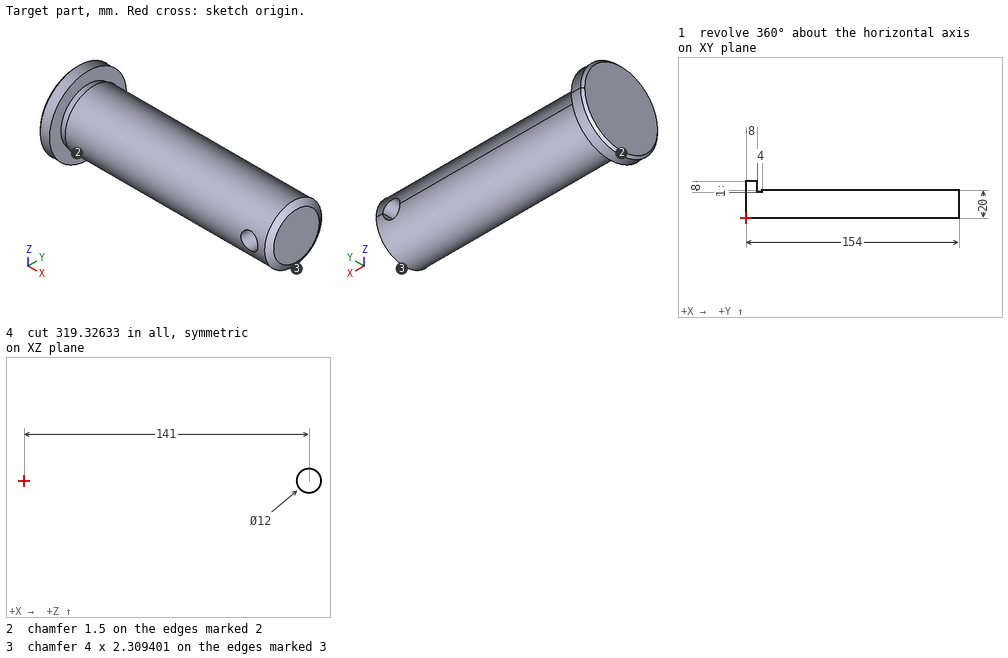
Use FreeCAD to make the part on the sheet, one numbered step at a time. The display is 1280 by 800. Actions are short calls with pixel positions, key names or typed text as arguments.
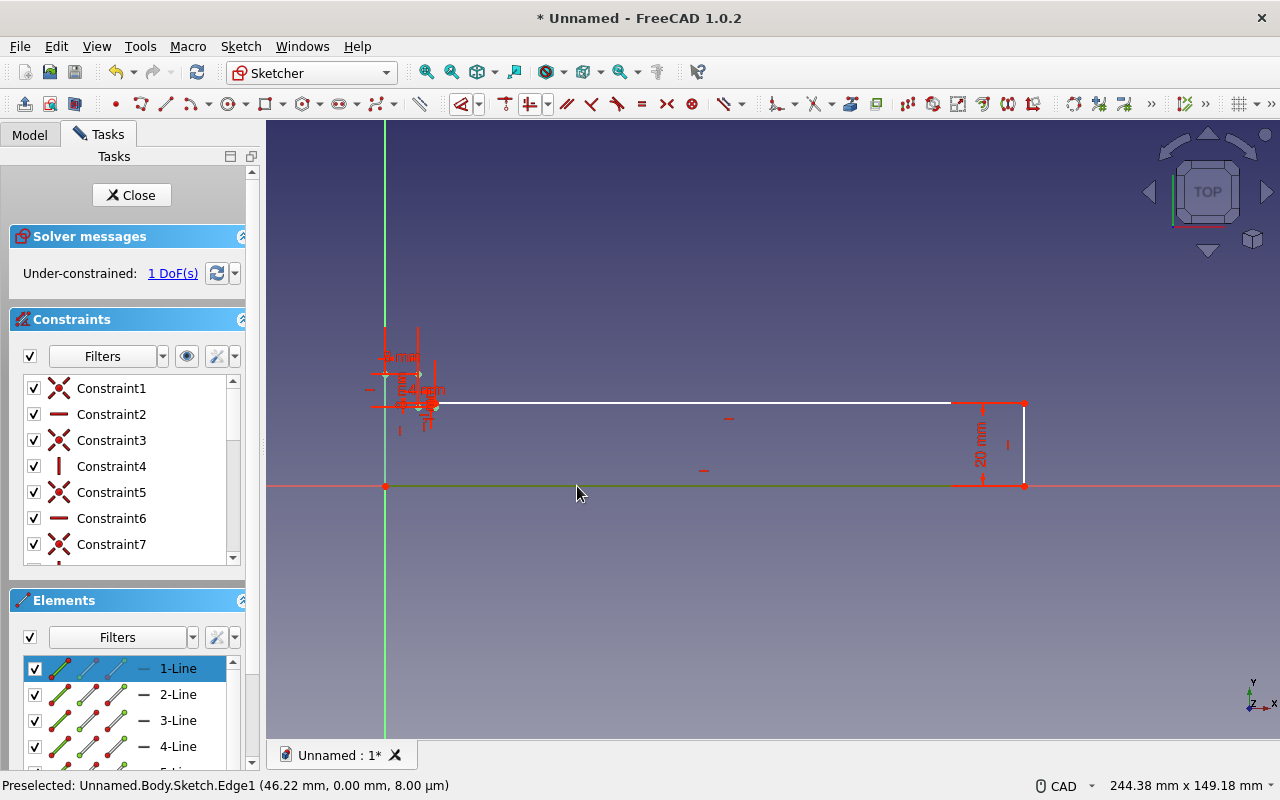
click(478, 104)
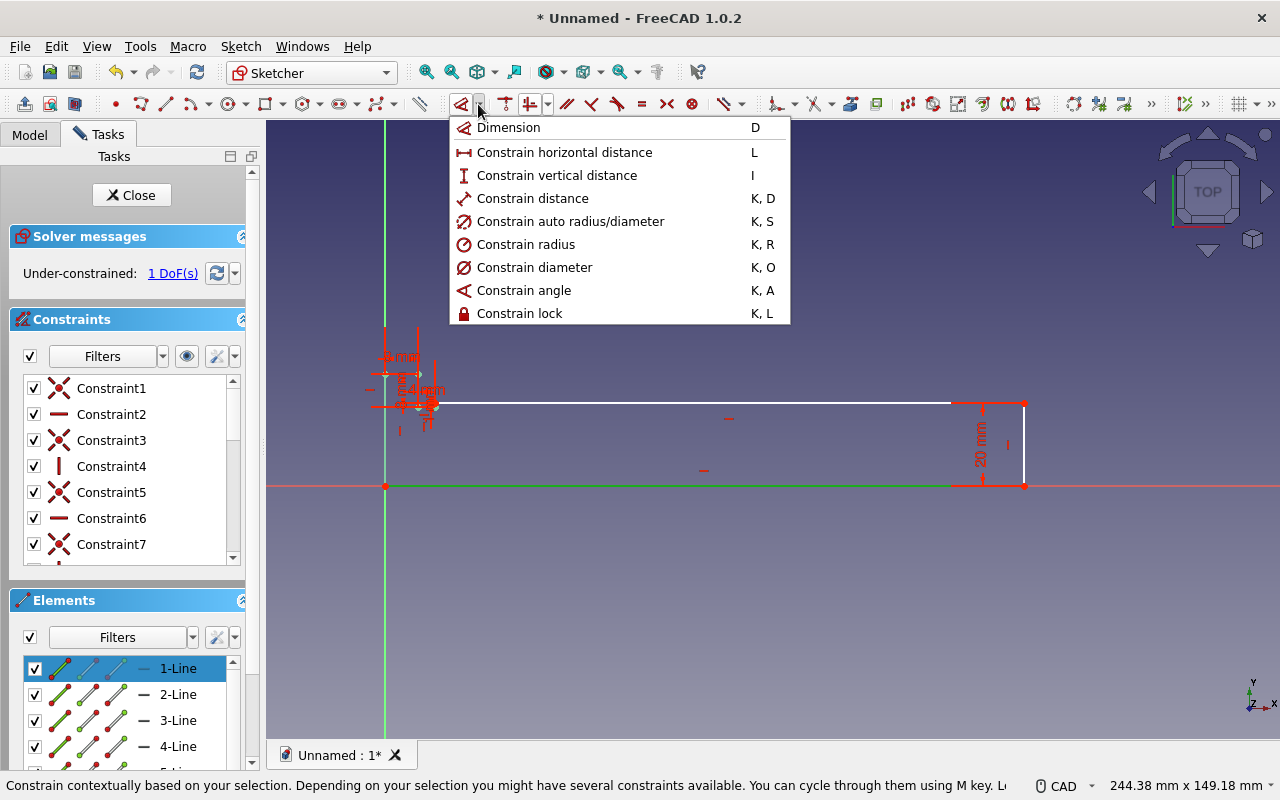
click(620, 152)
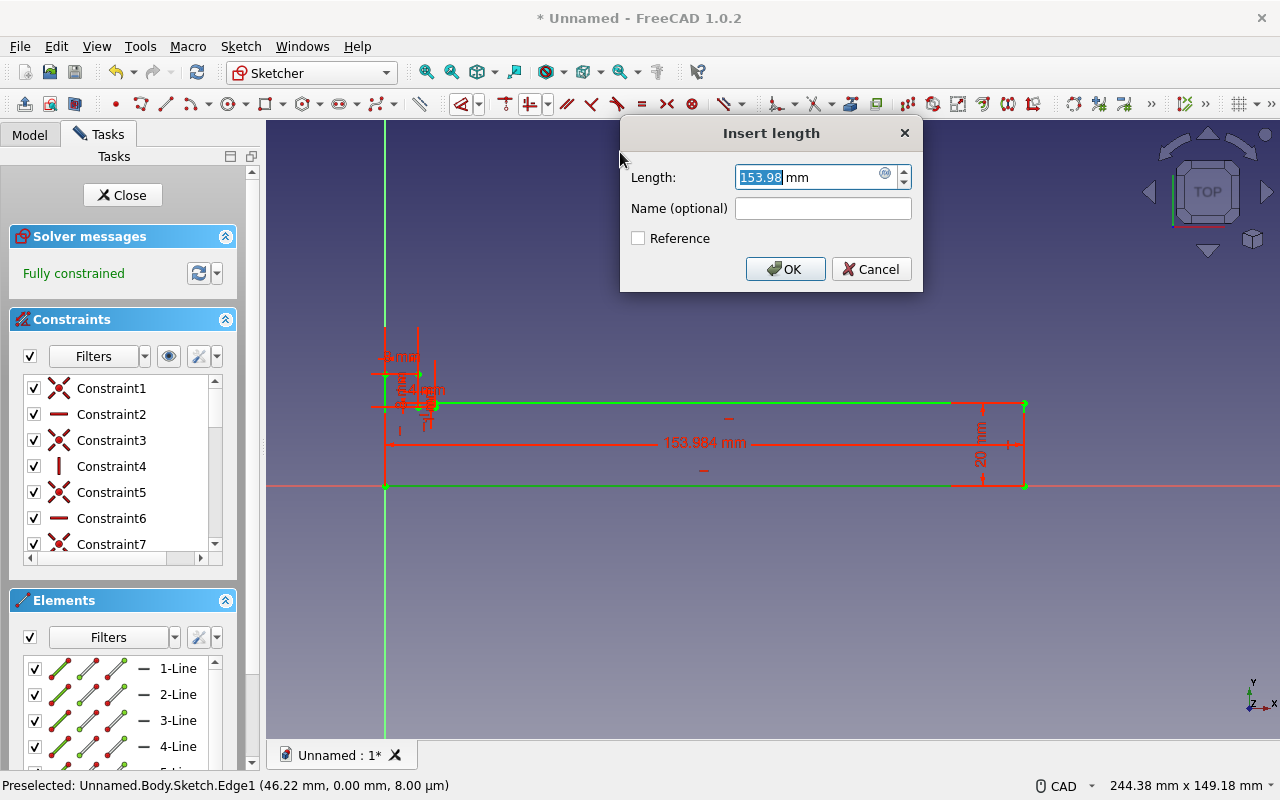
text(154)
key(Return)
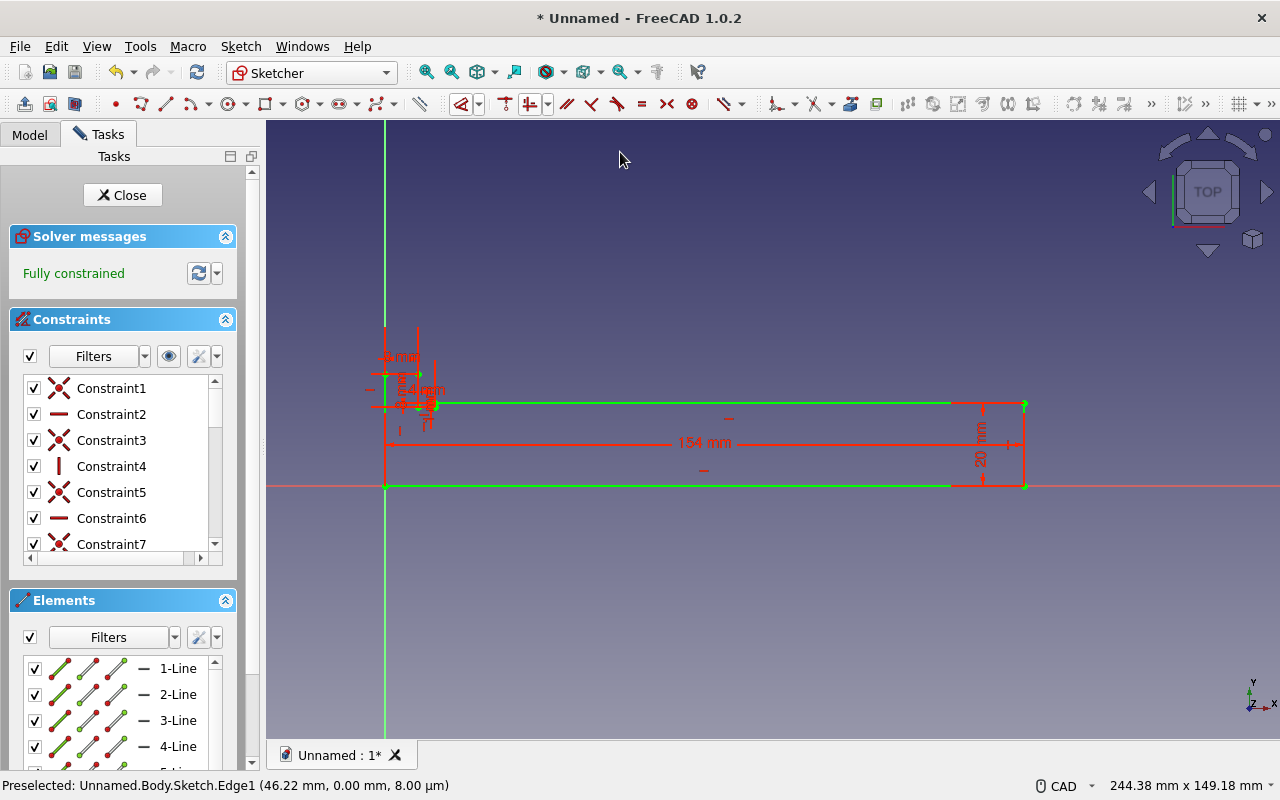
click(123, 195)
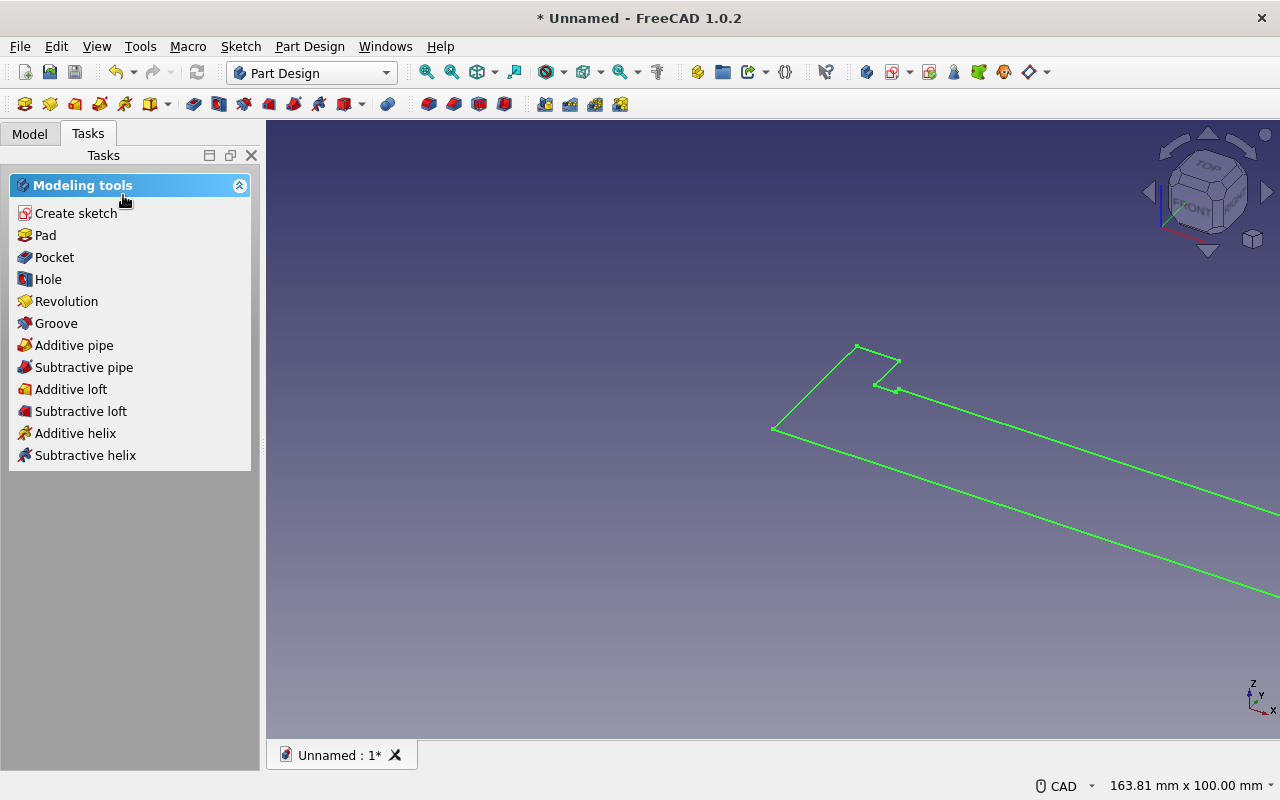
click(50, 104)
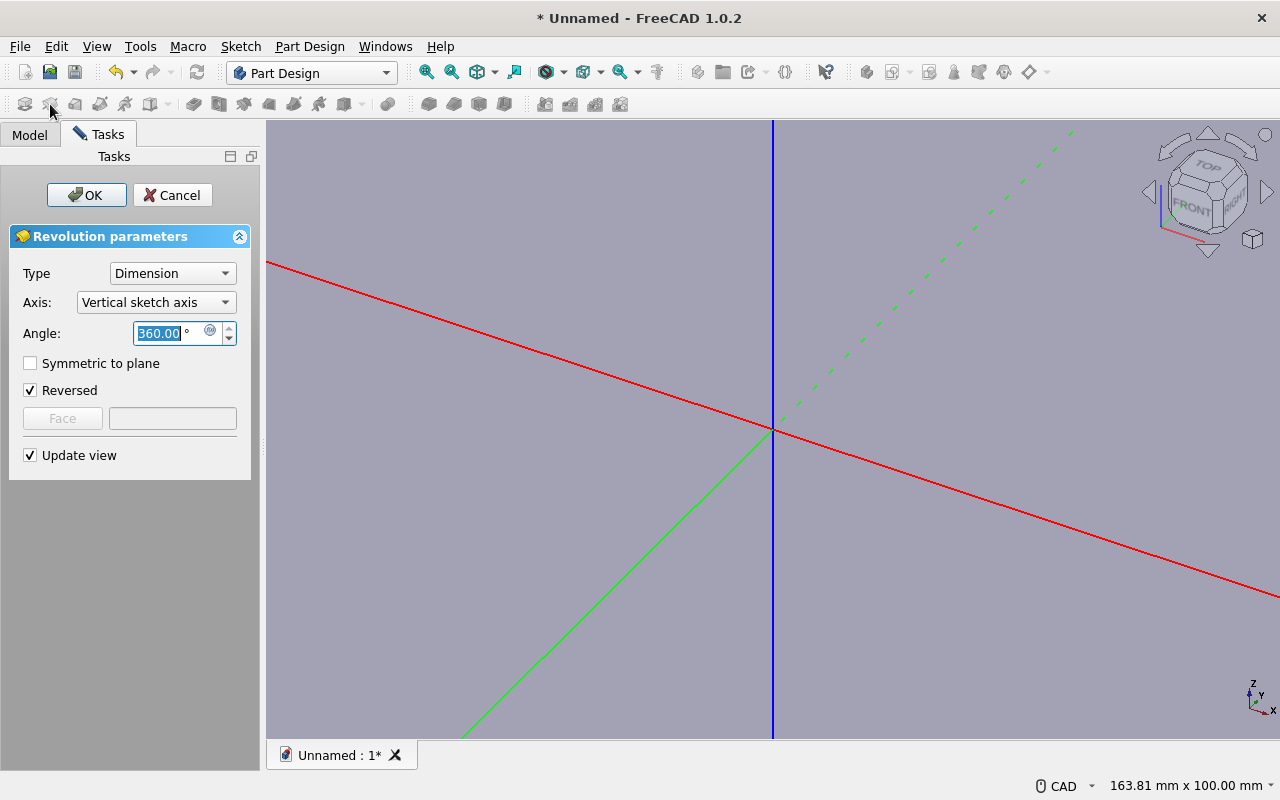
click(157, 302)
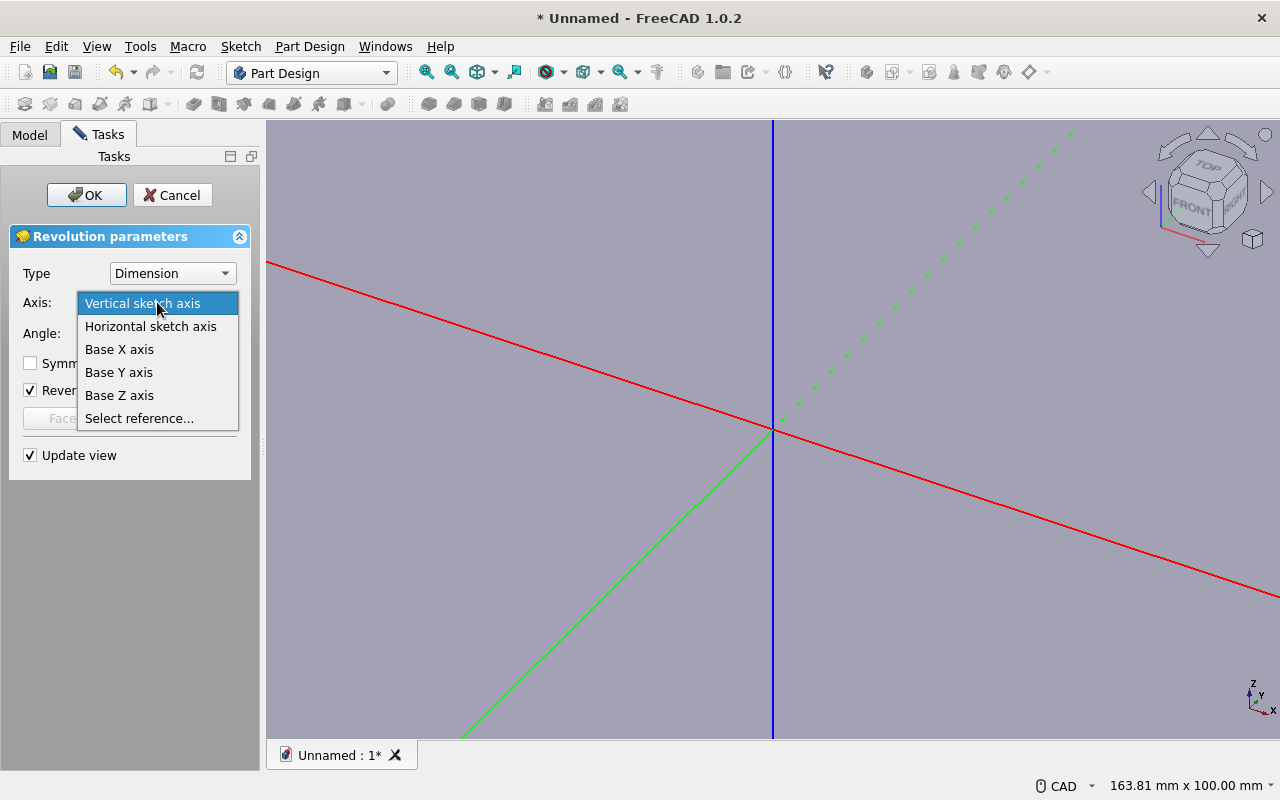
click(156, 326)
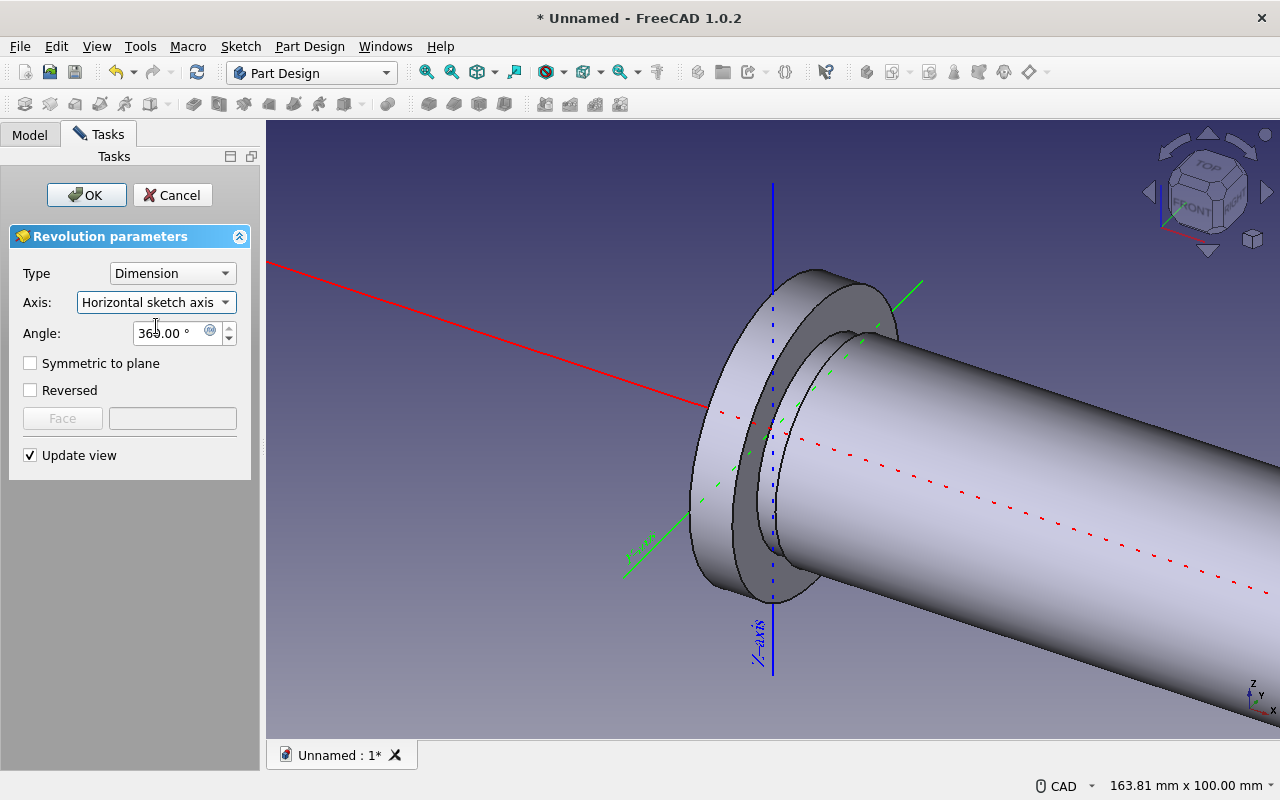
click(87, 195)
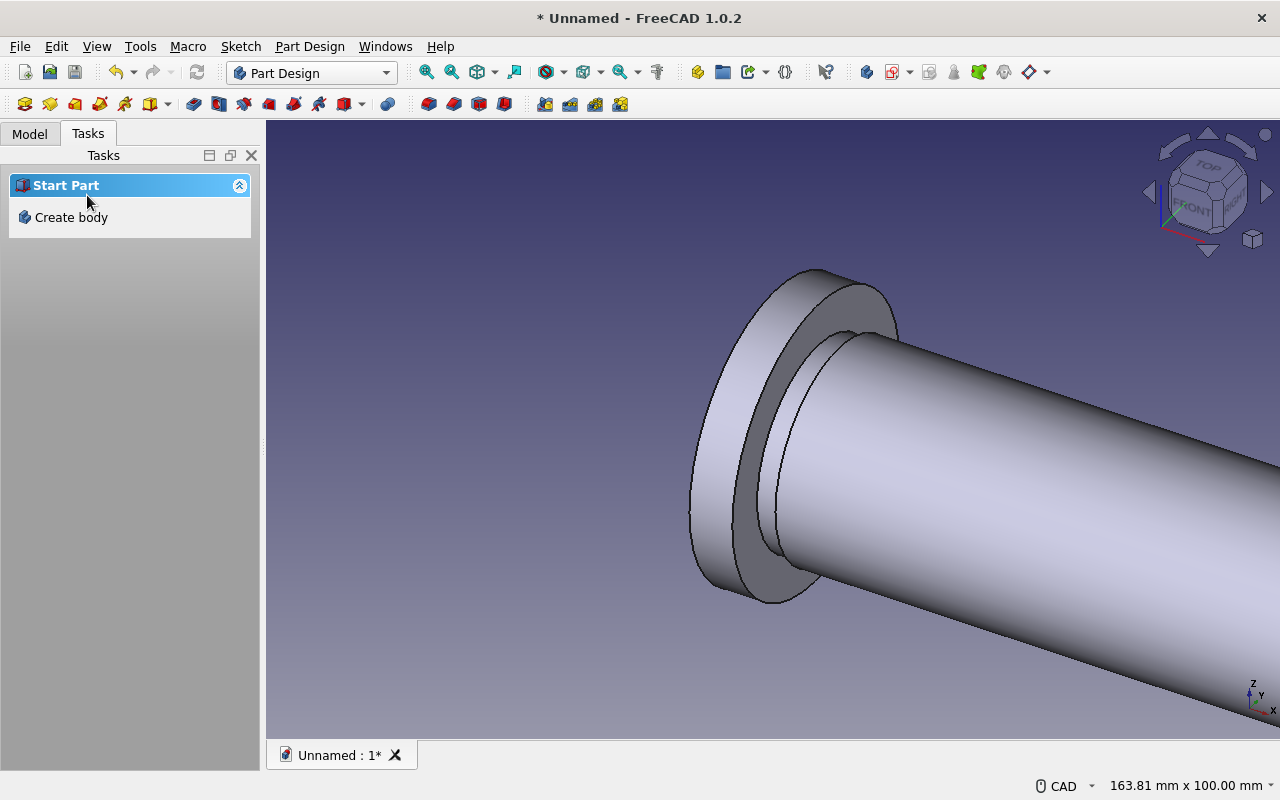
click(427, 72)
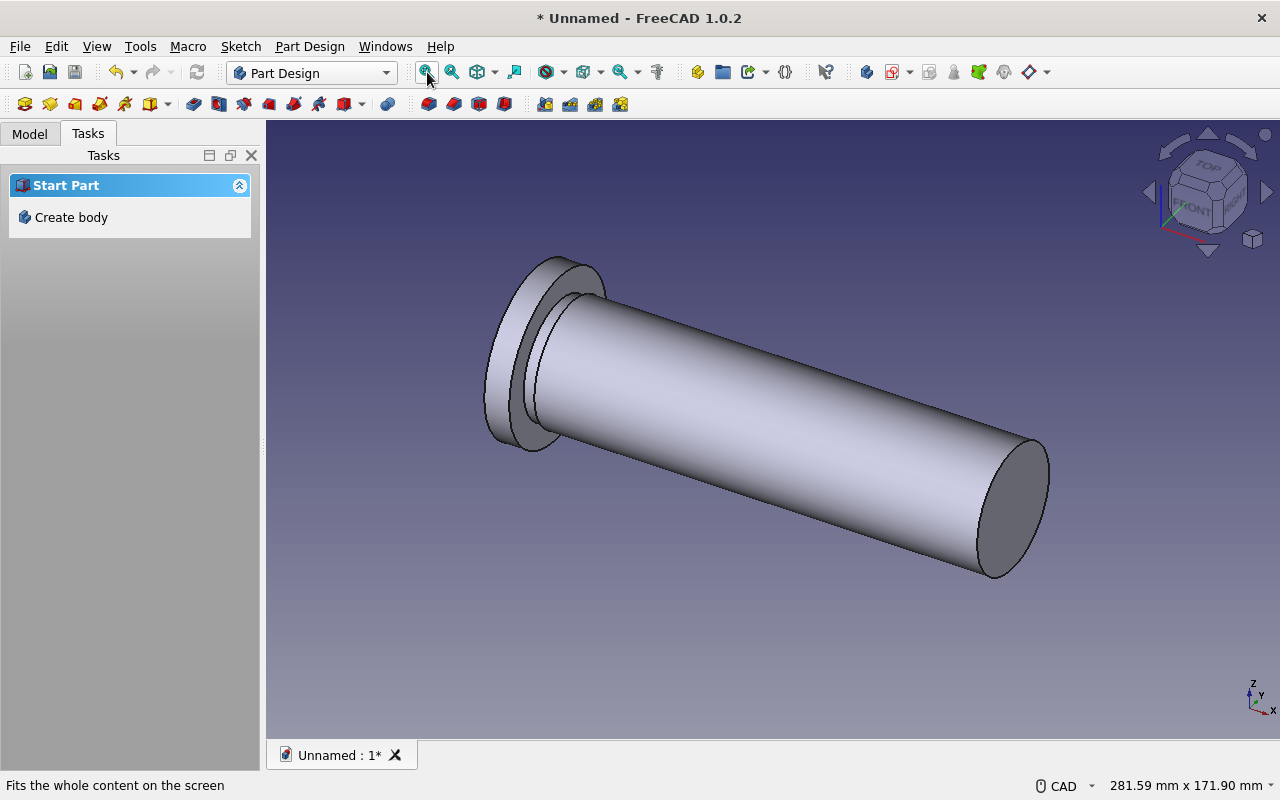
key(0)